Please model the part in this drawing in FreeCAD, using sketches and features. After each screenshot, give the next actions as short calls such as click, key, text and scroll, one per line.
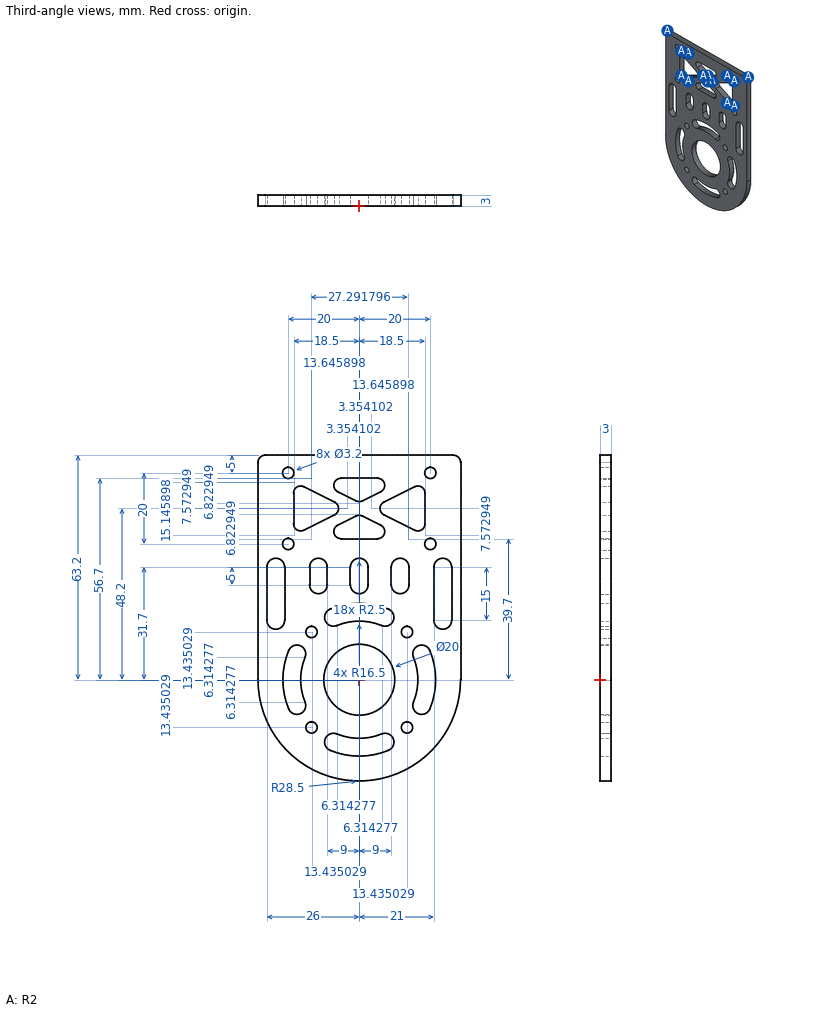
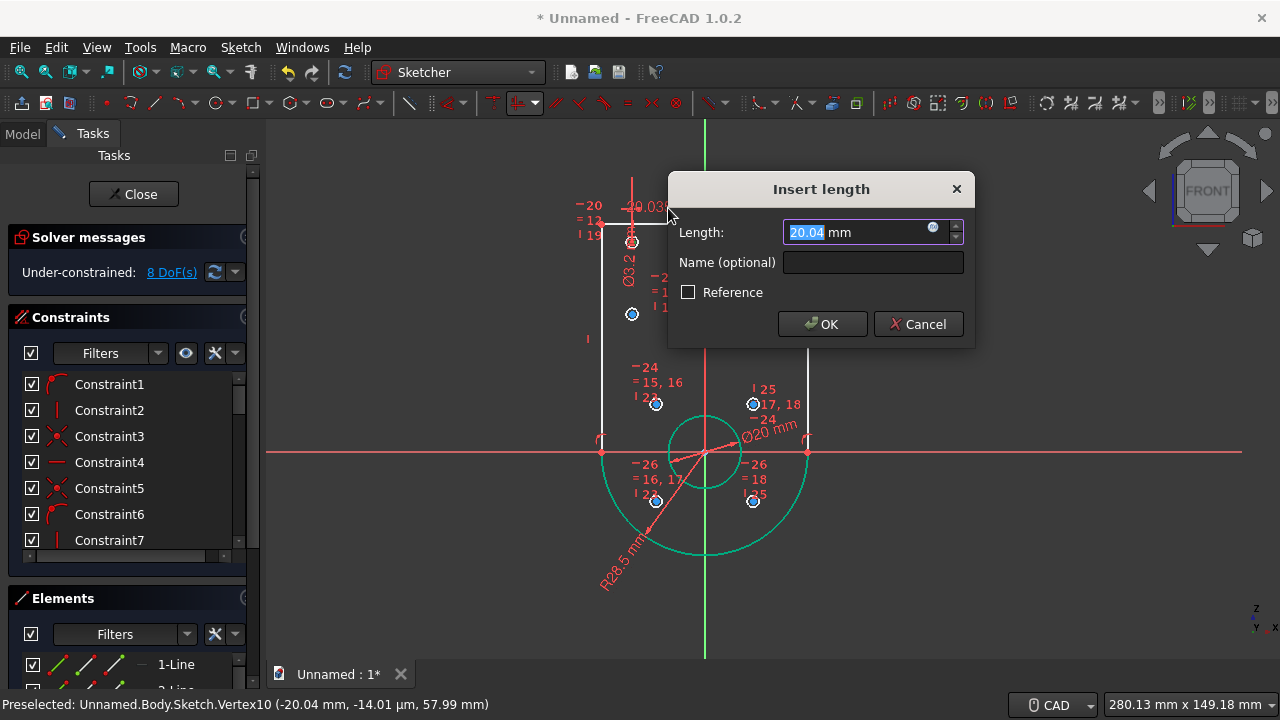
text(20)
key(Return)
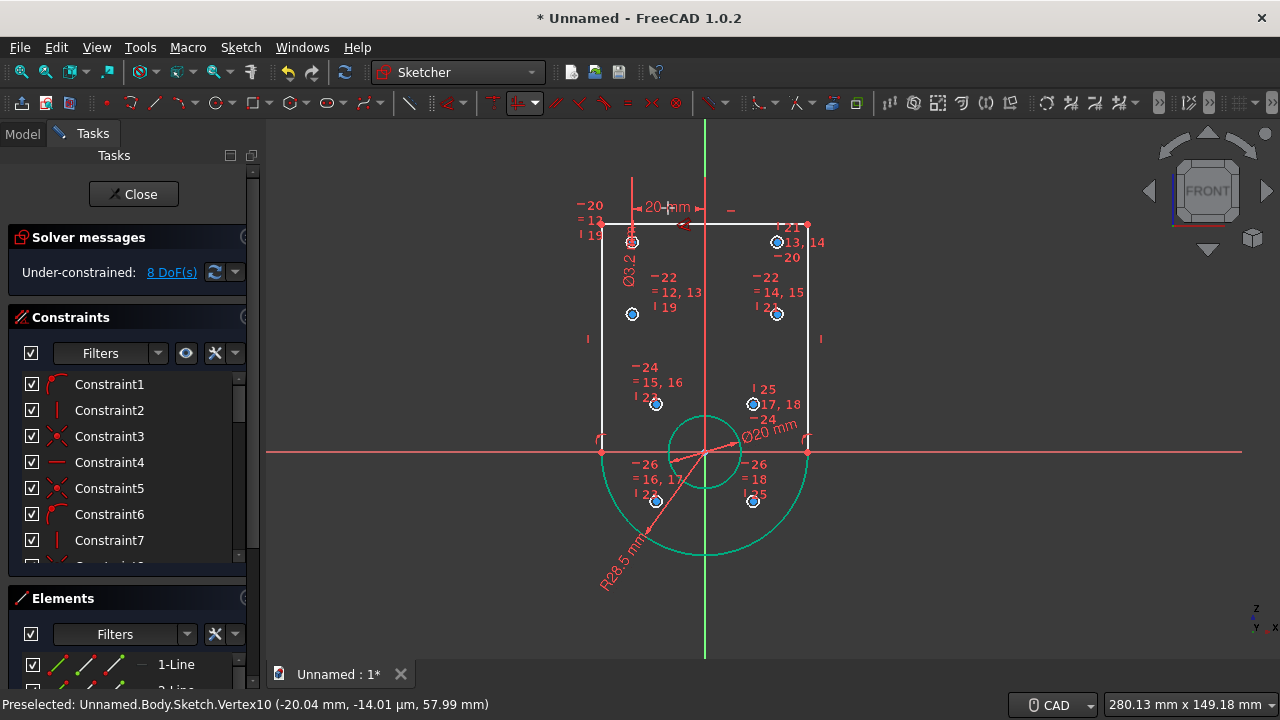
click(777, 242)
click(741, 208)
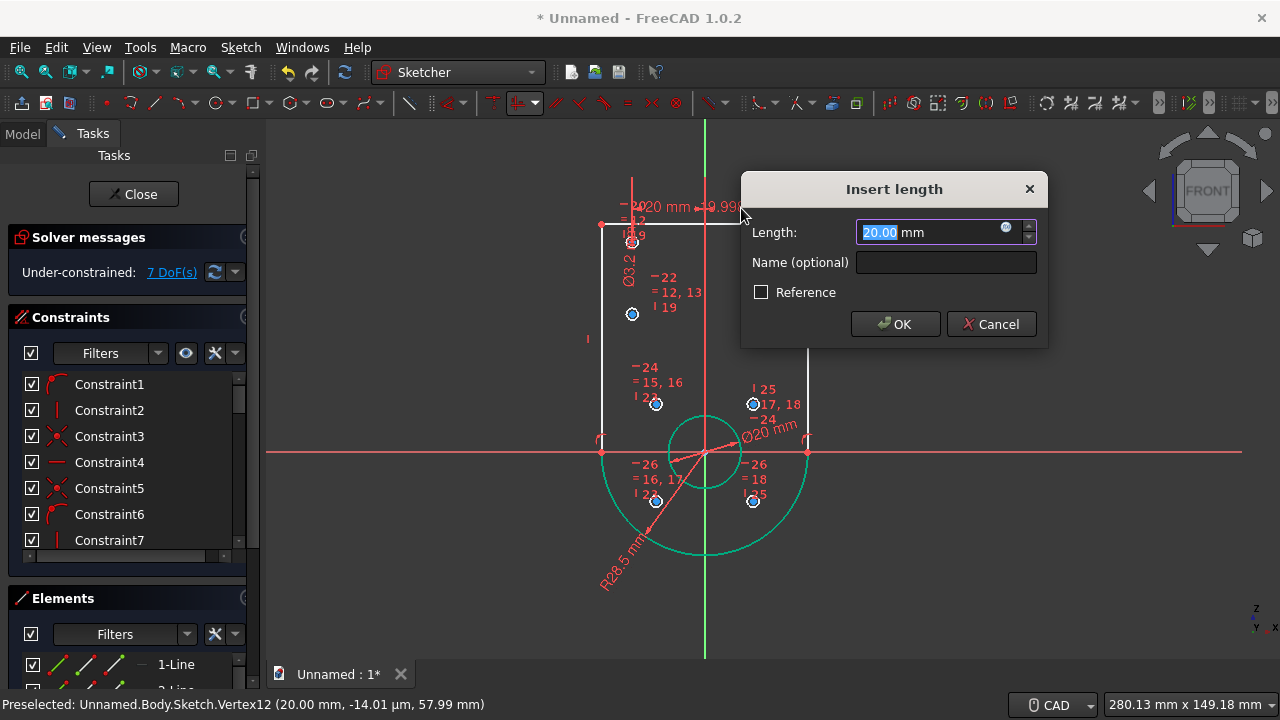
text(20)
key(Return)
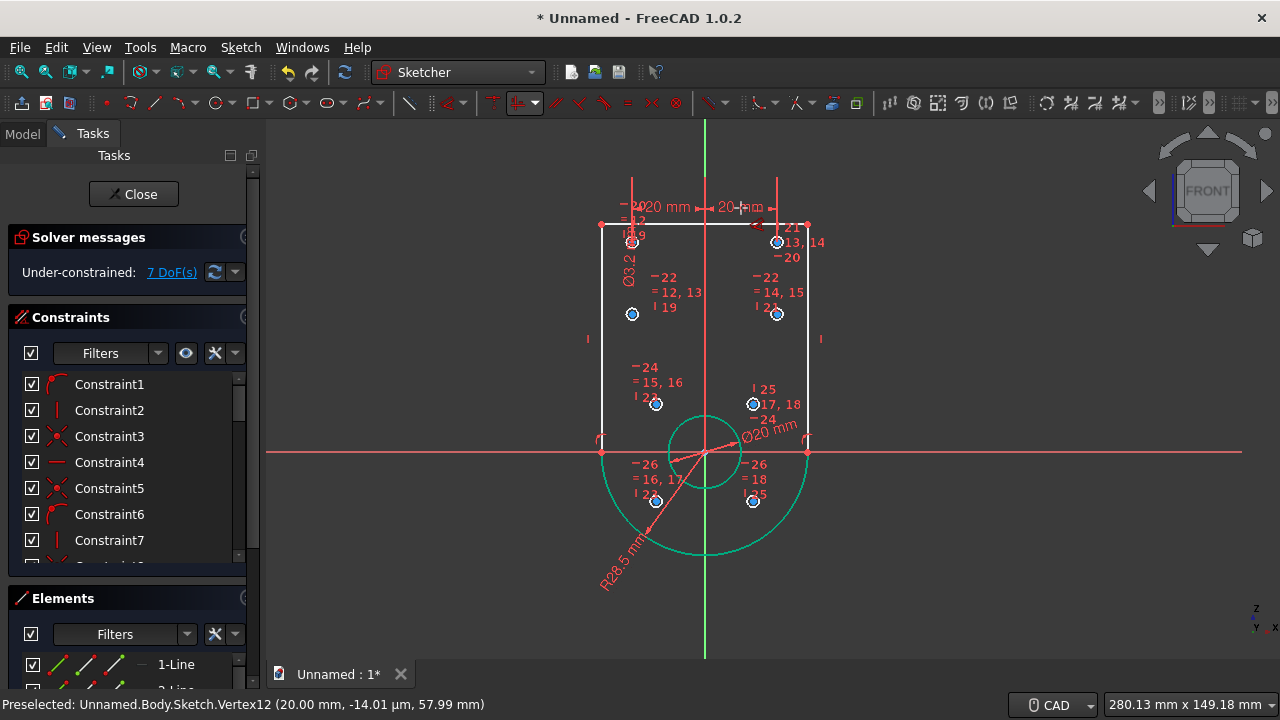
scroll(602, 224, up, 4)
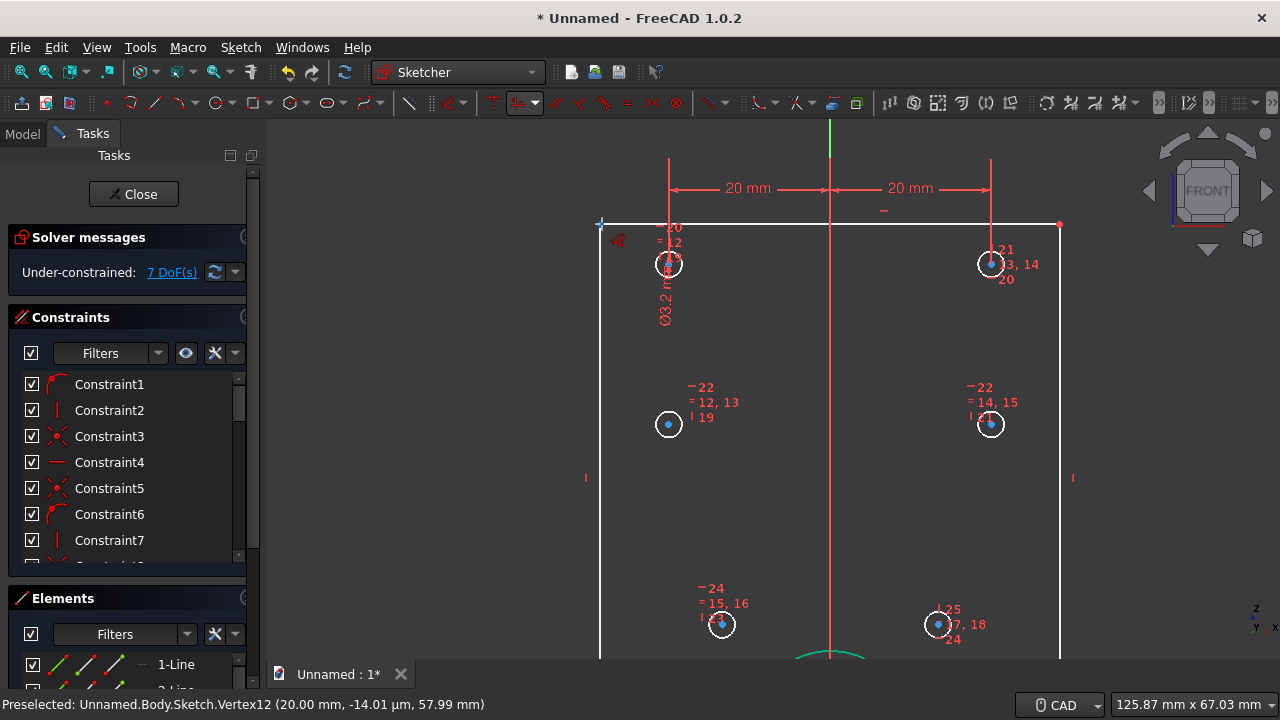
click(600, 224)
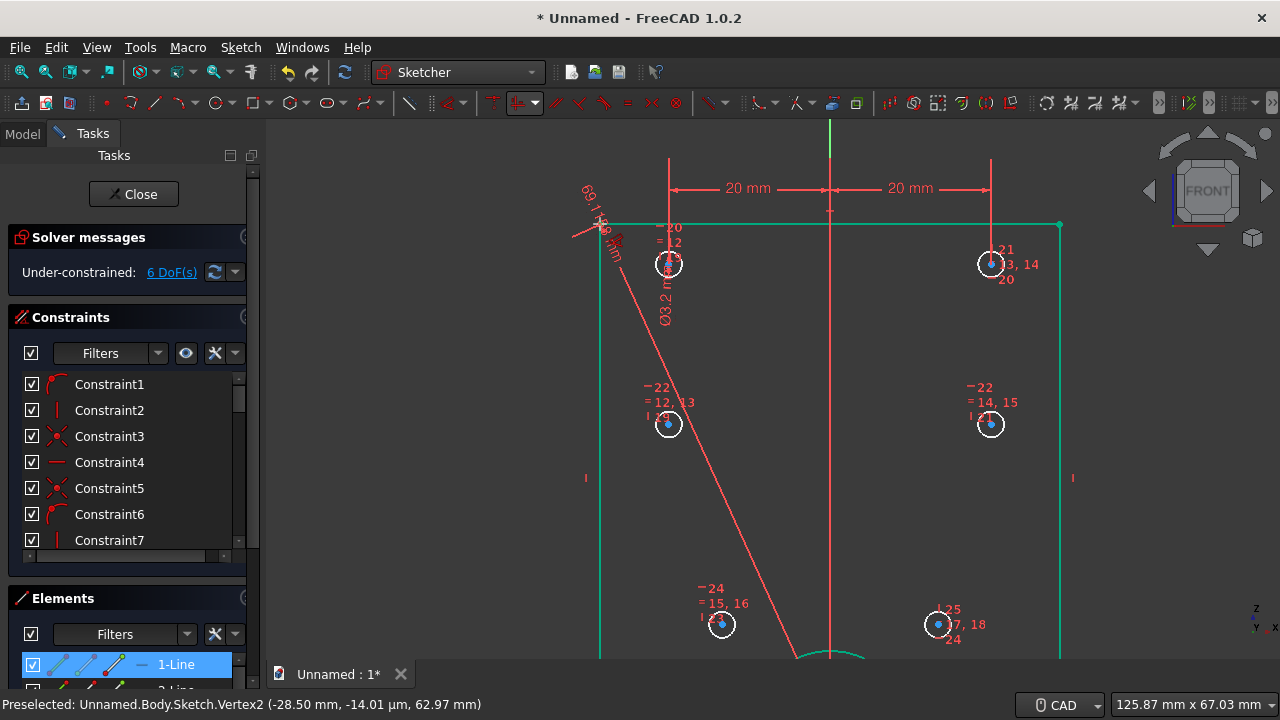
click(669, 264)
click(566, 244)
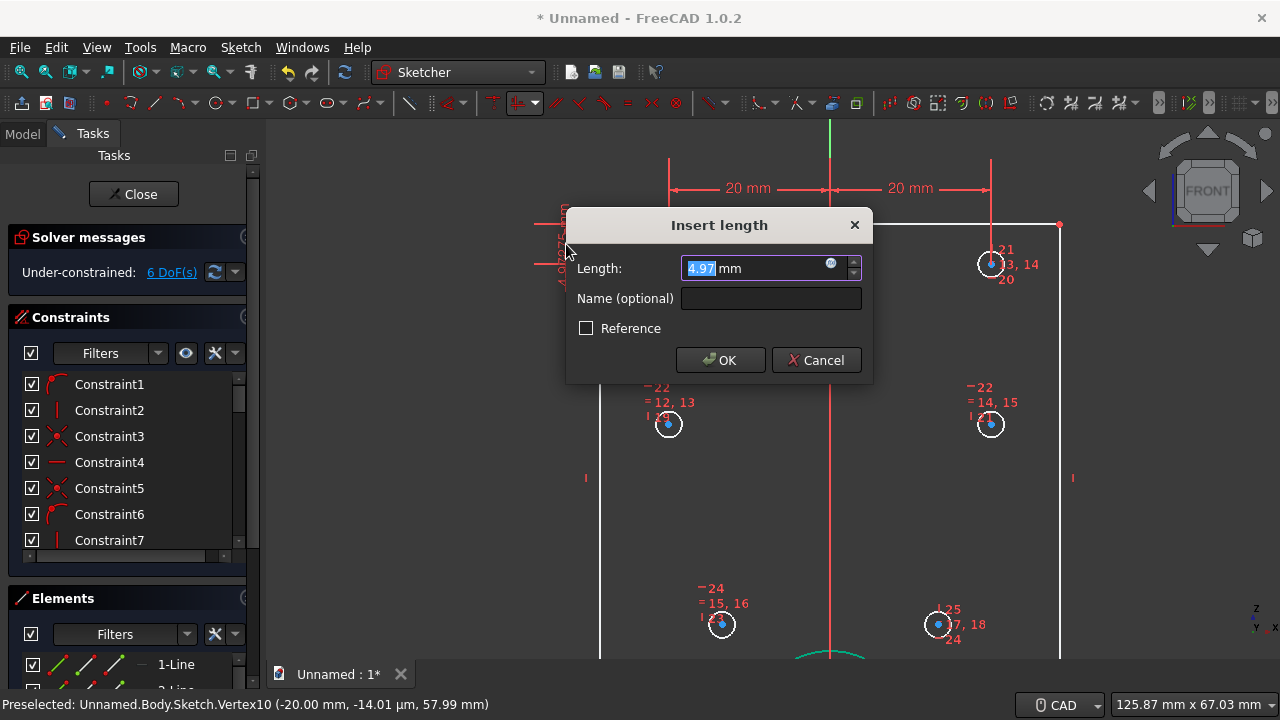
text(5)
key(Return)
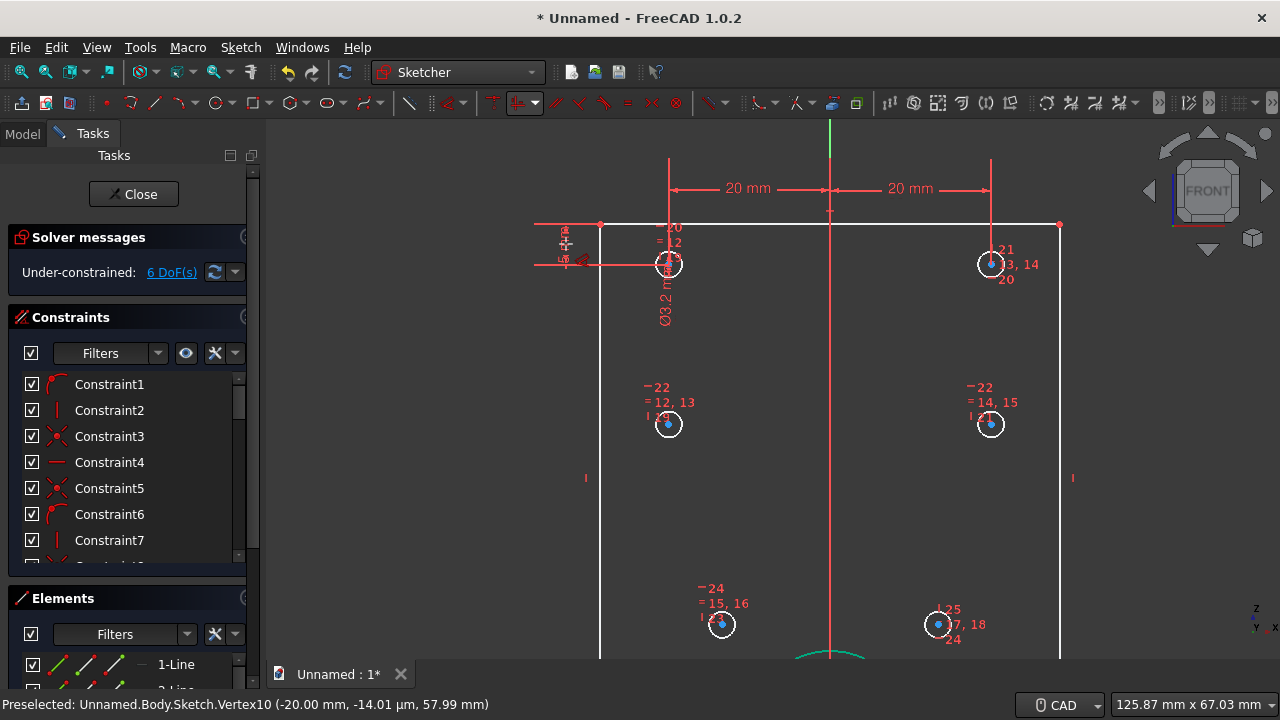
click(669, 265)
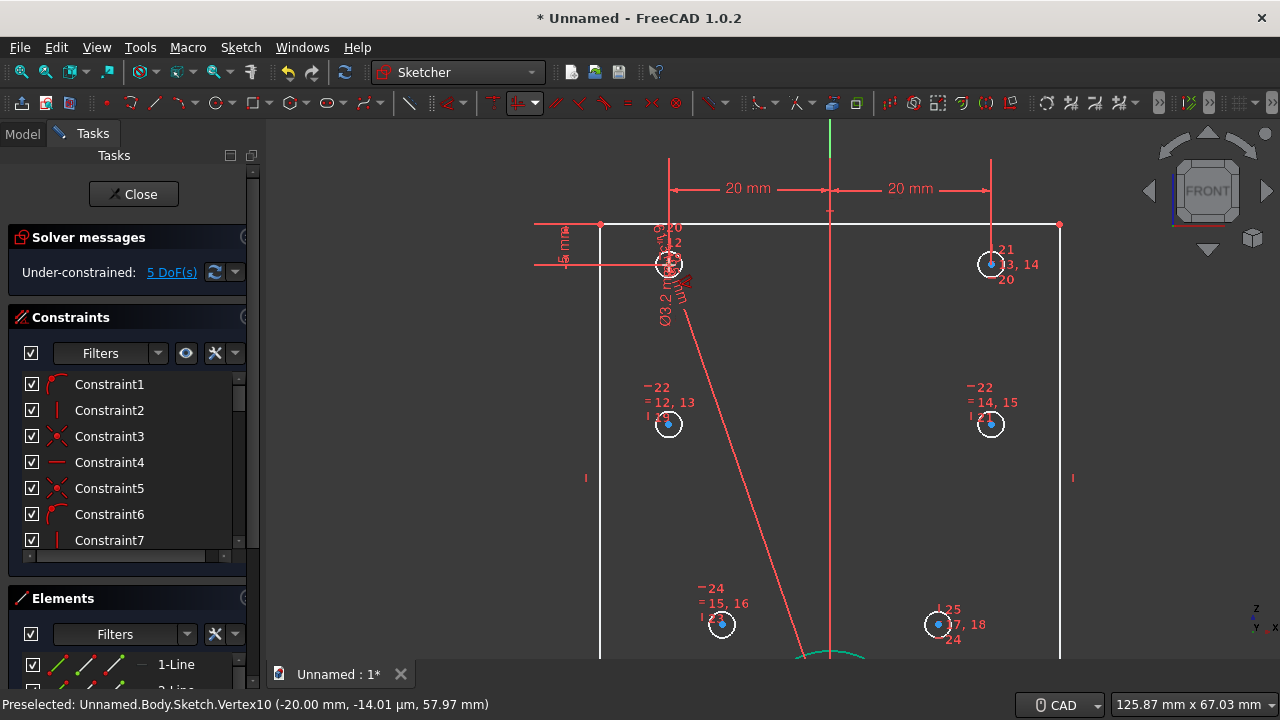
click(669, 424)
click(635, 345)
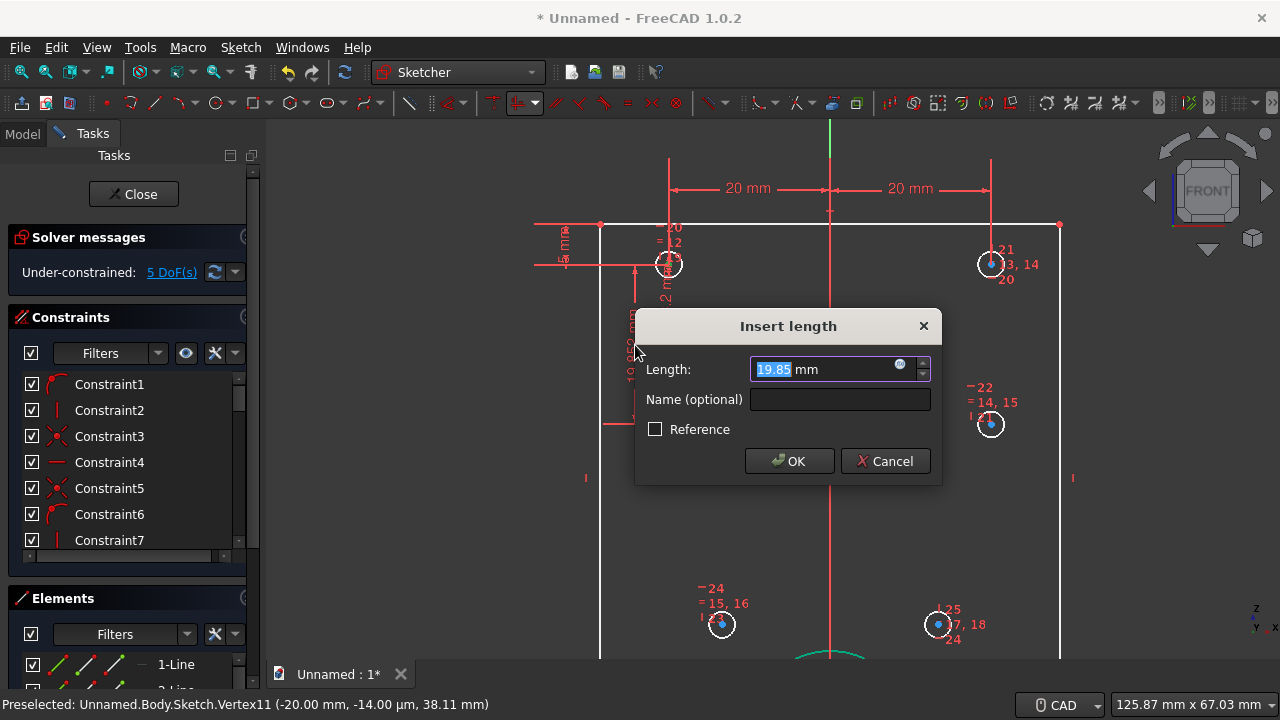
text(20)
key(Return)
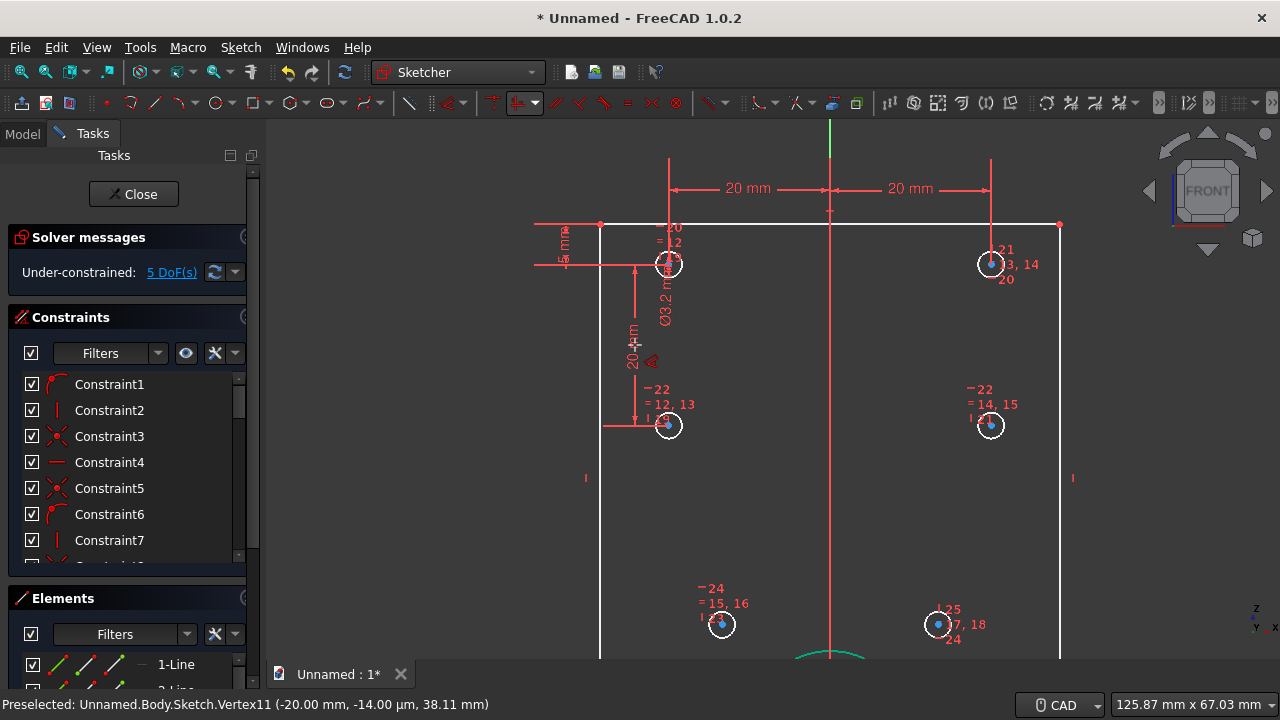
click(600, 579)
click(566, 428)